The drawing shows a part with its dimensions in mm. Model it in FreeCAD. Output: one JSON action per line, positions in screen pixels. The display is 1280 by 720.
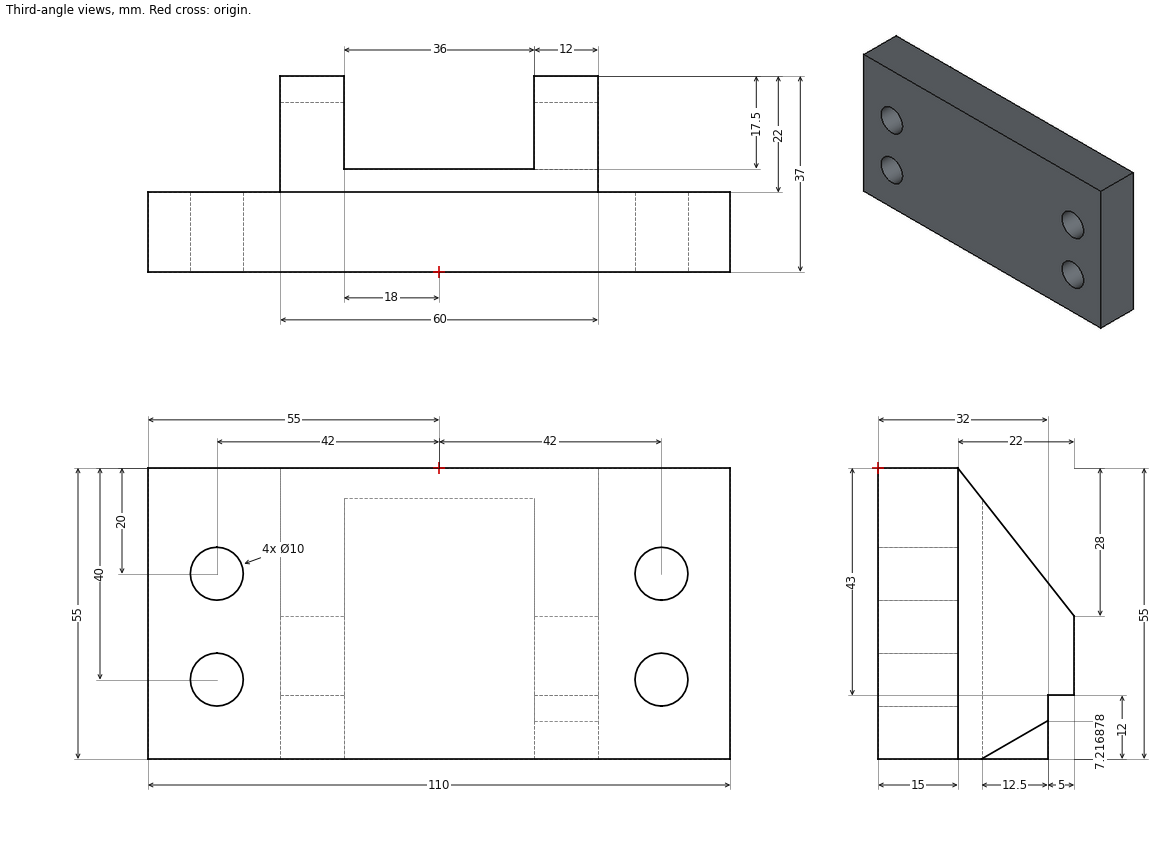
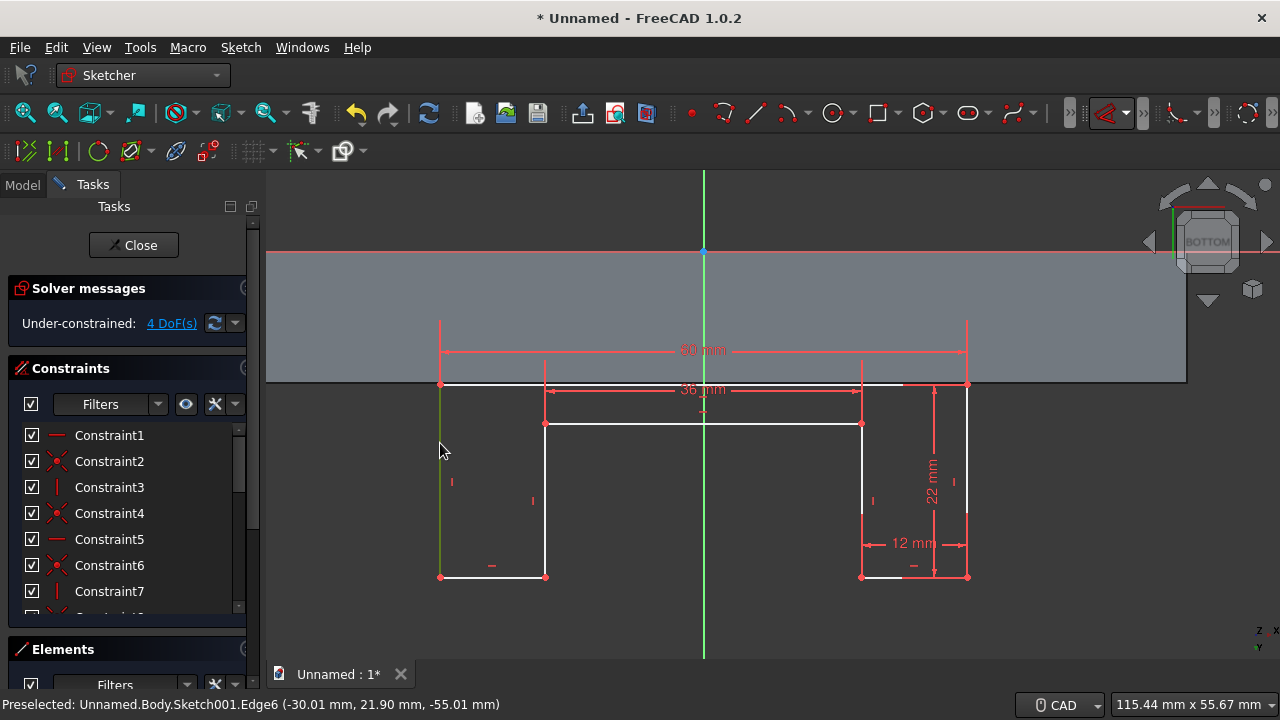
{"action": "key", "text": "i"}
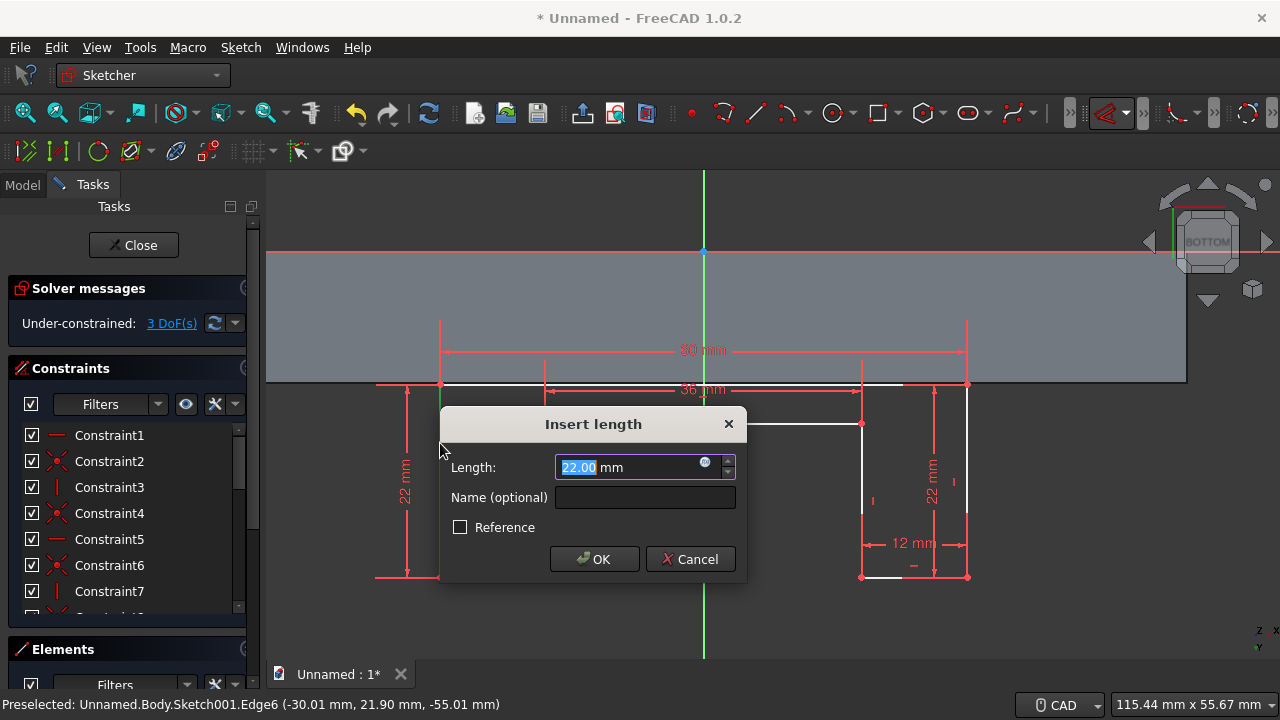
{"action": "type", "text": "22"}
{"action": "key", "text": "Return"}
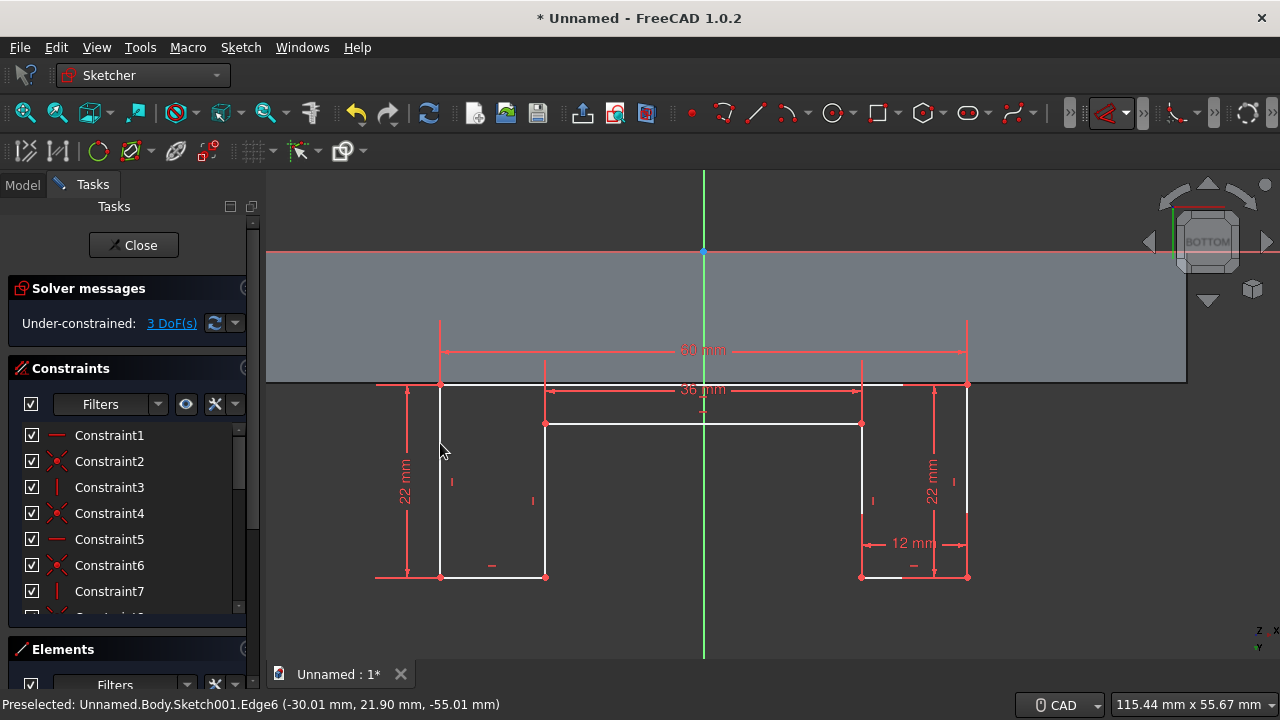
{"action": "left_click", "coordinate": [545, 424]}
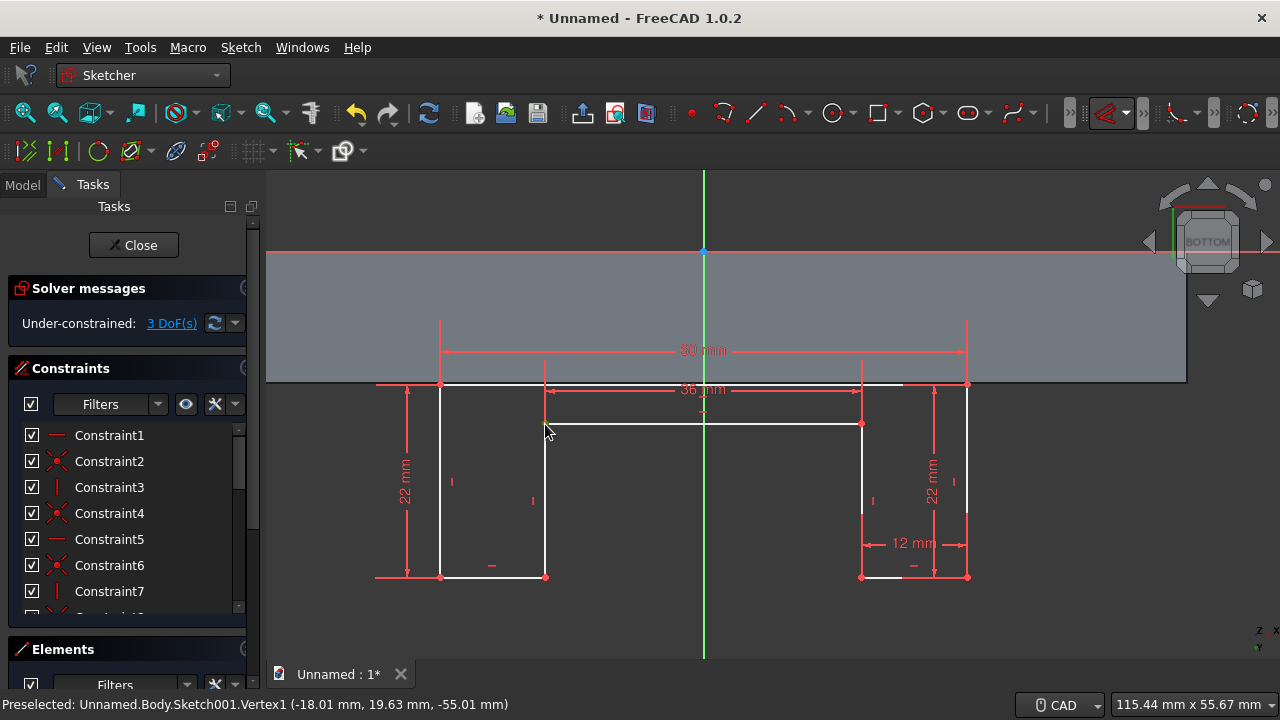
{"action": "key", "text": "l"}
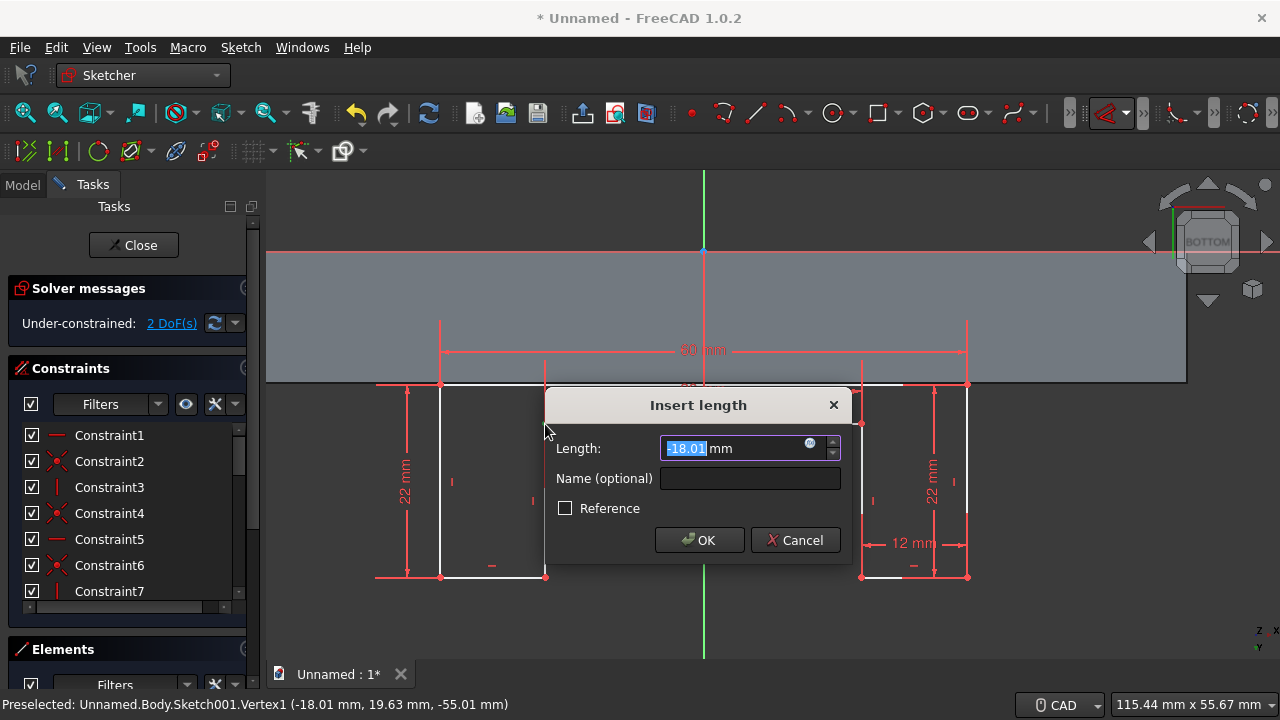
{"action": "type", "text": "-18"}
{"action": "key", "text": "Return"}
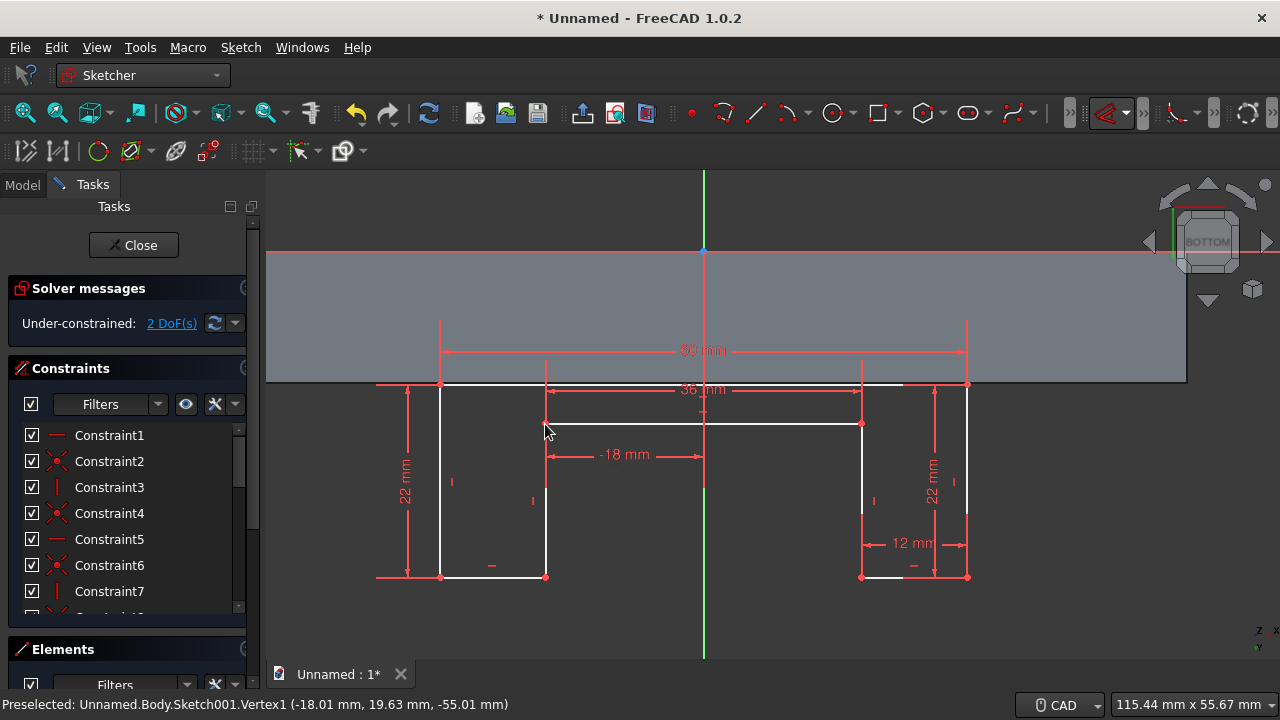
{"action": "left_click", "coordinate": [862, 578]}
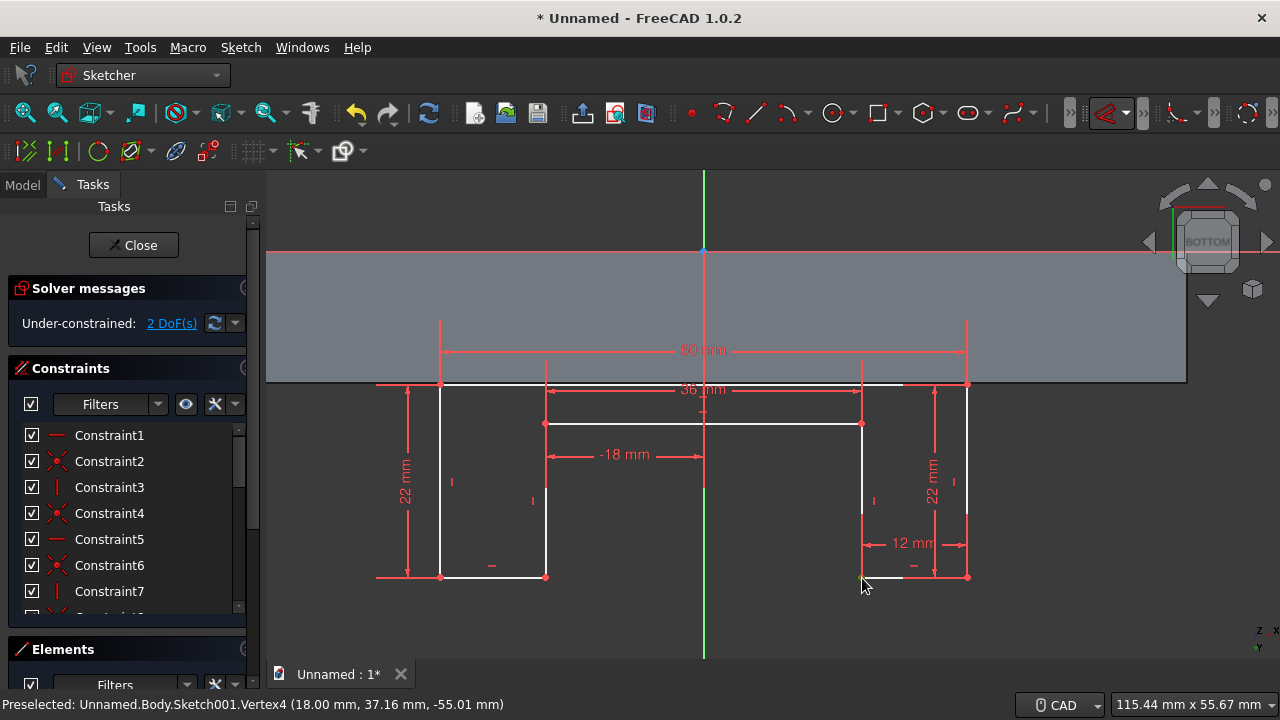
{"action": "key", "text": "i"}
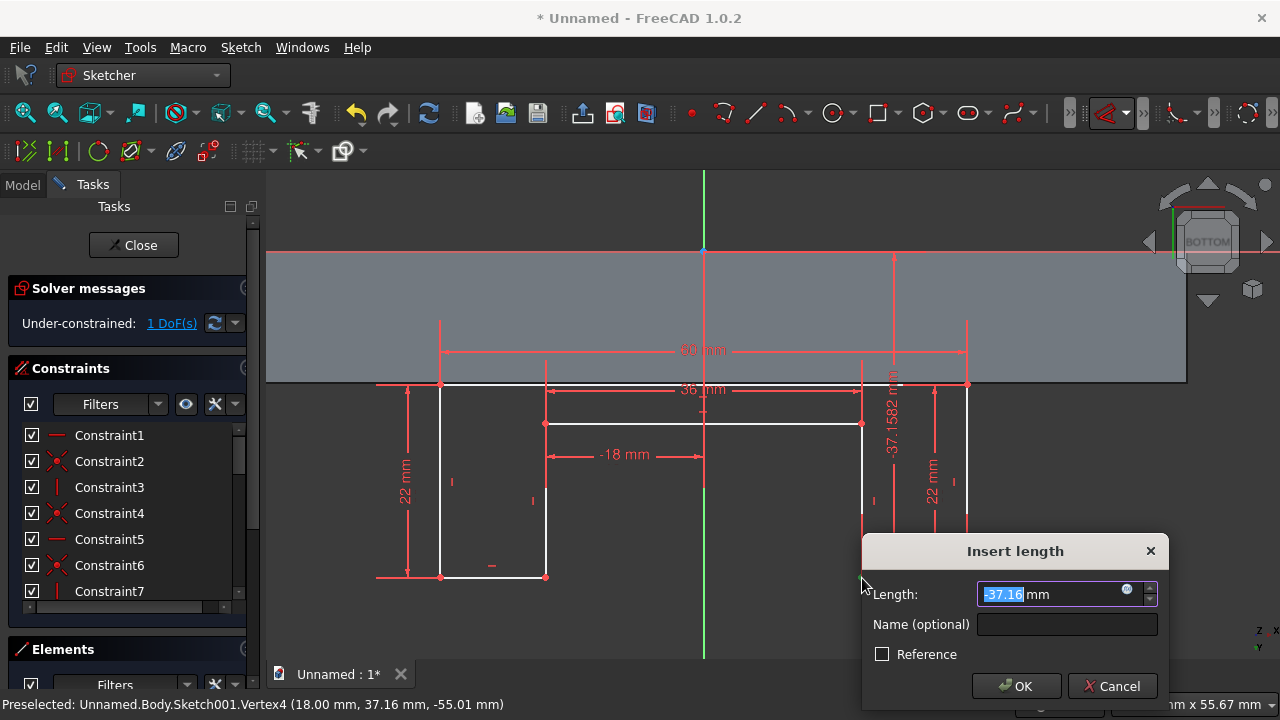
{"action": "type", "text": "-37"}
{"action": "key", "text": "Return"}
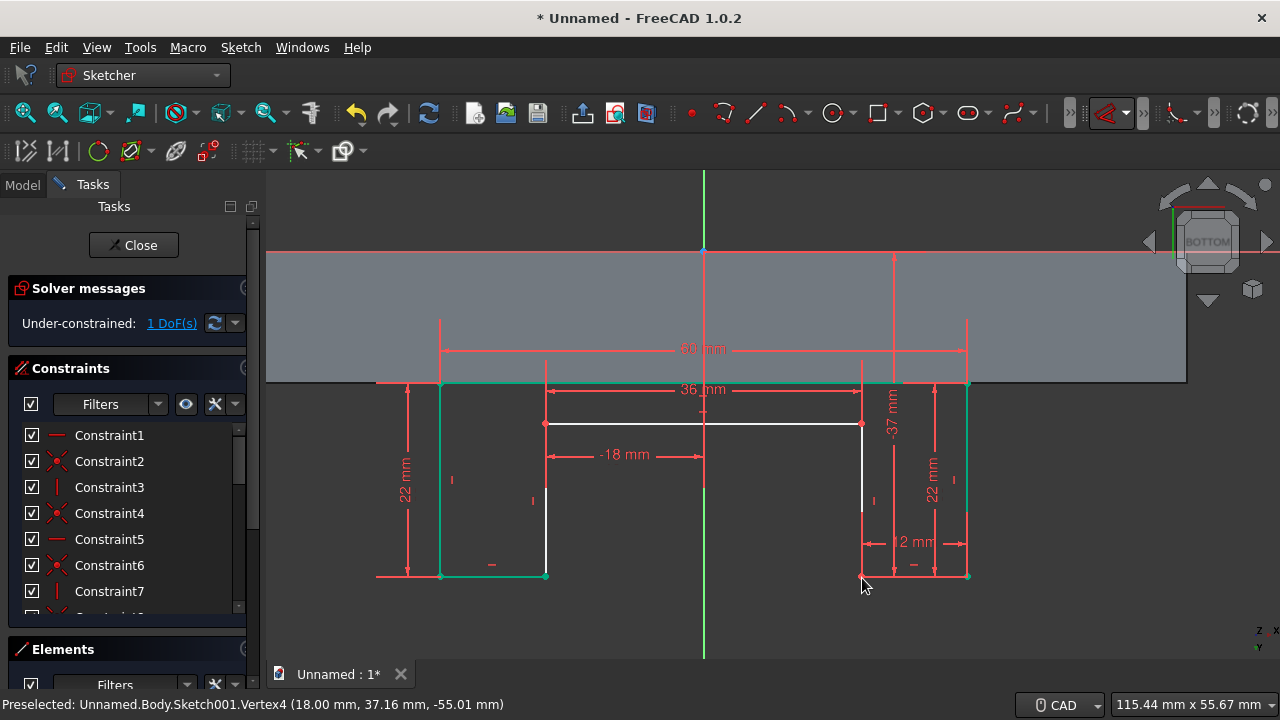
{"action": "left_click", "coordinate": [862, 470]}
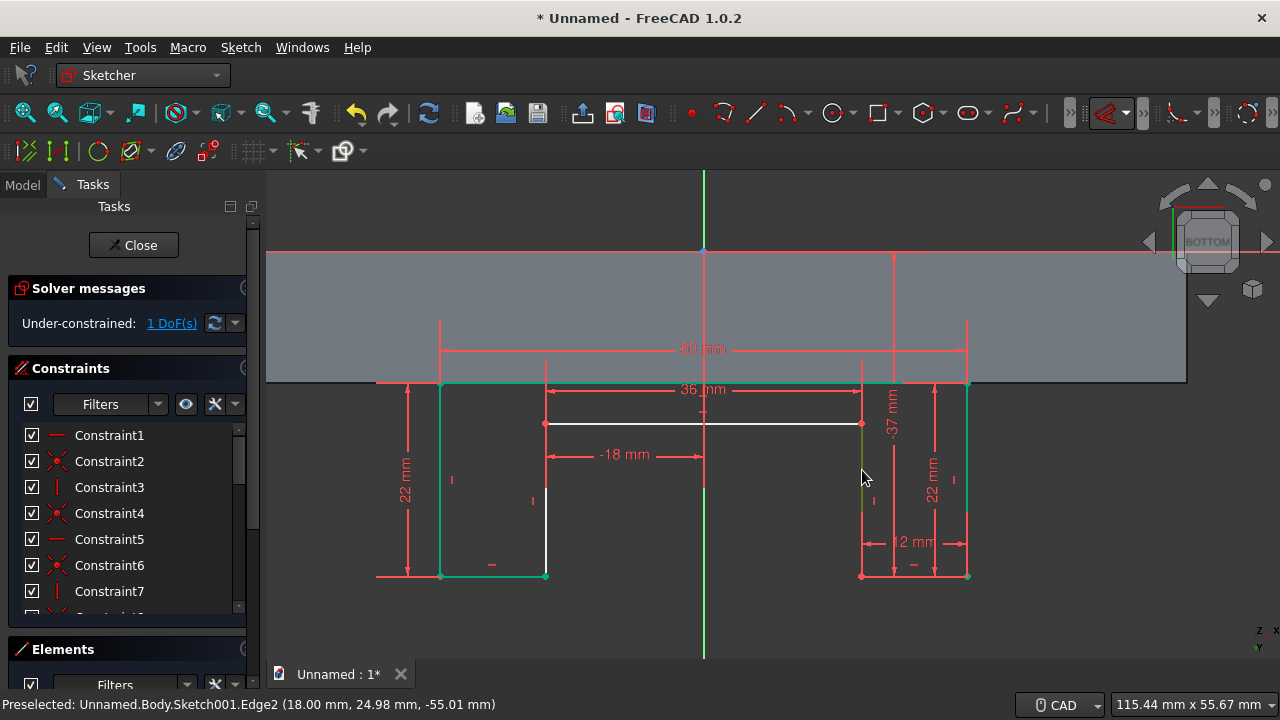
{"action": "key", "text": "i"}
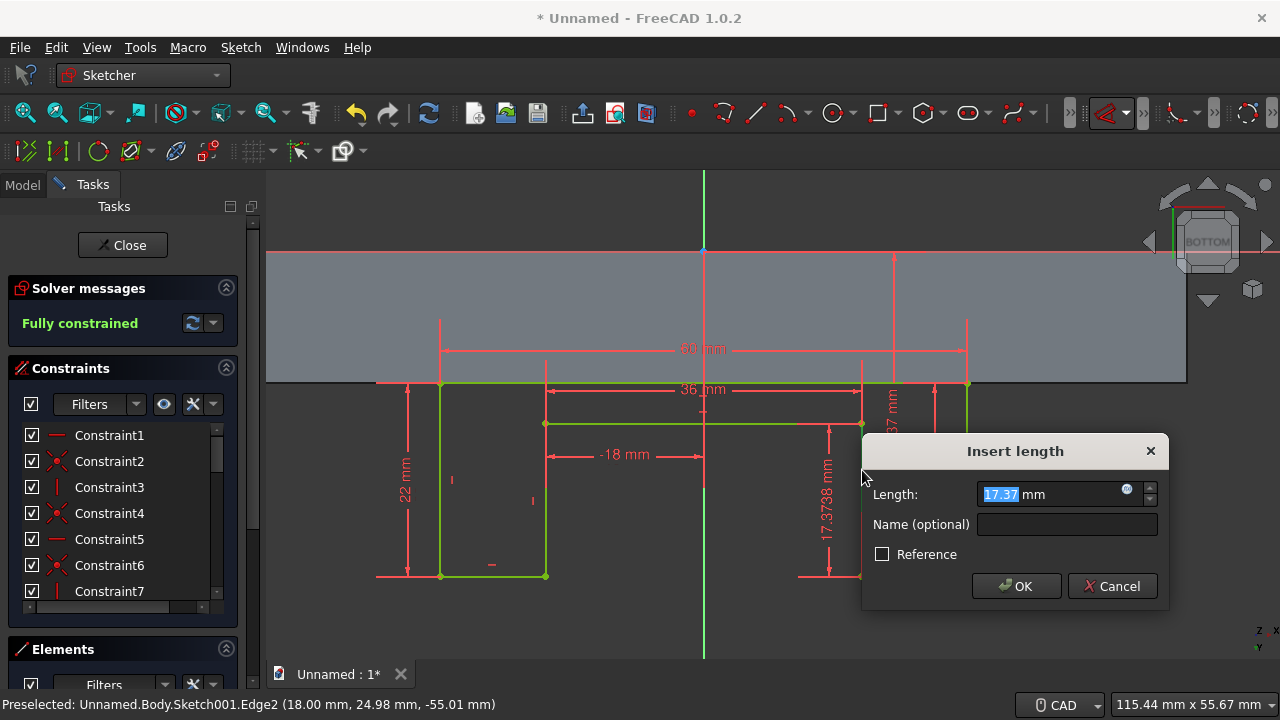
{"action": "type", "text": "17.5"}
{"action": "key", "text": "Return"}